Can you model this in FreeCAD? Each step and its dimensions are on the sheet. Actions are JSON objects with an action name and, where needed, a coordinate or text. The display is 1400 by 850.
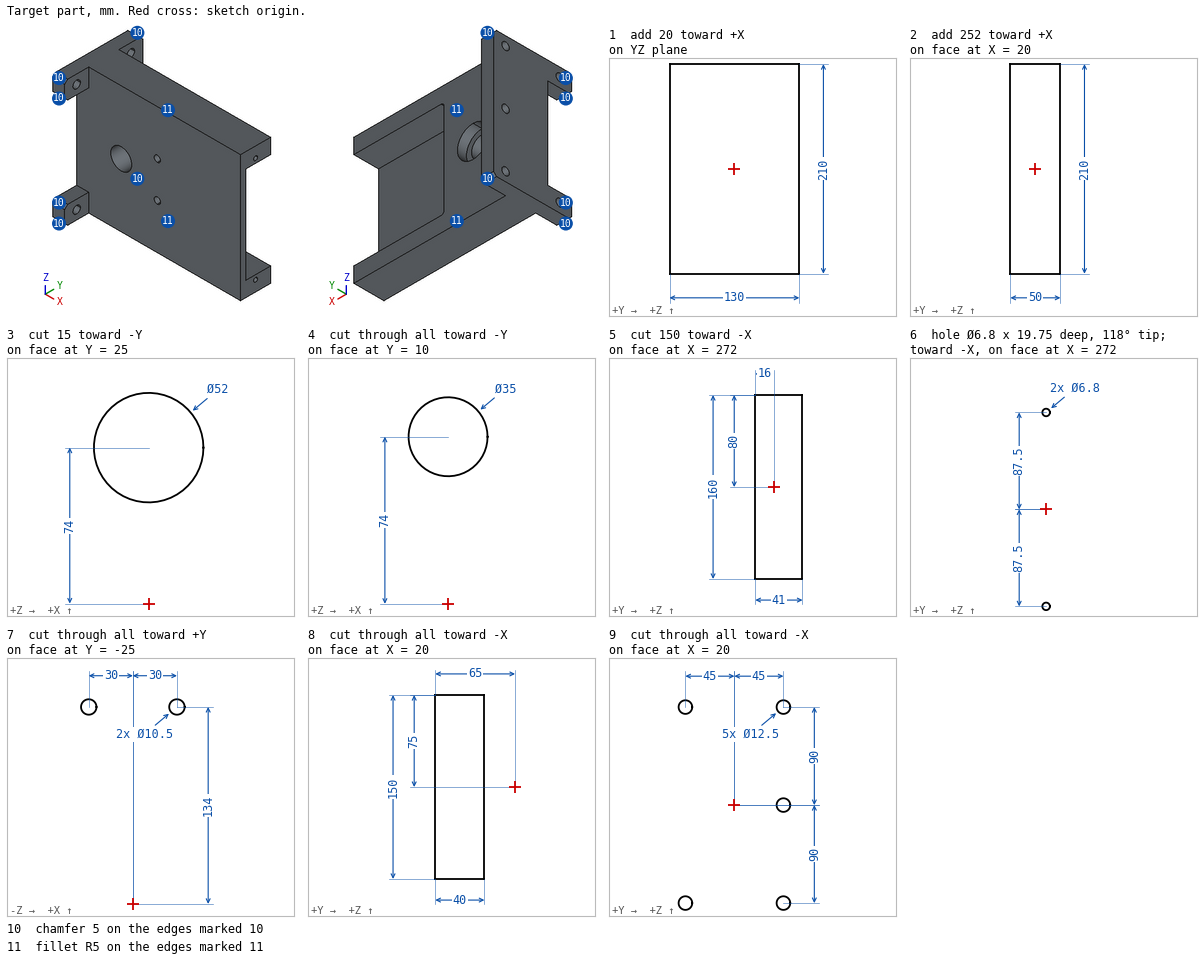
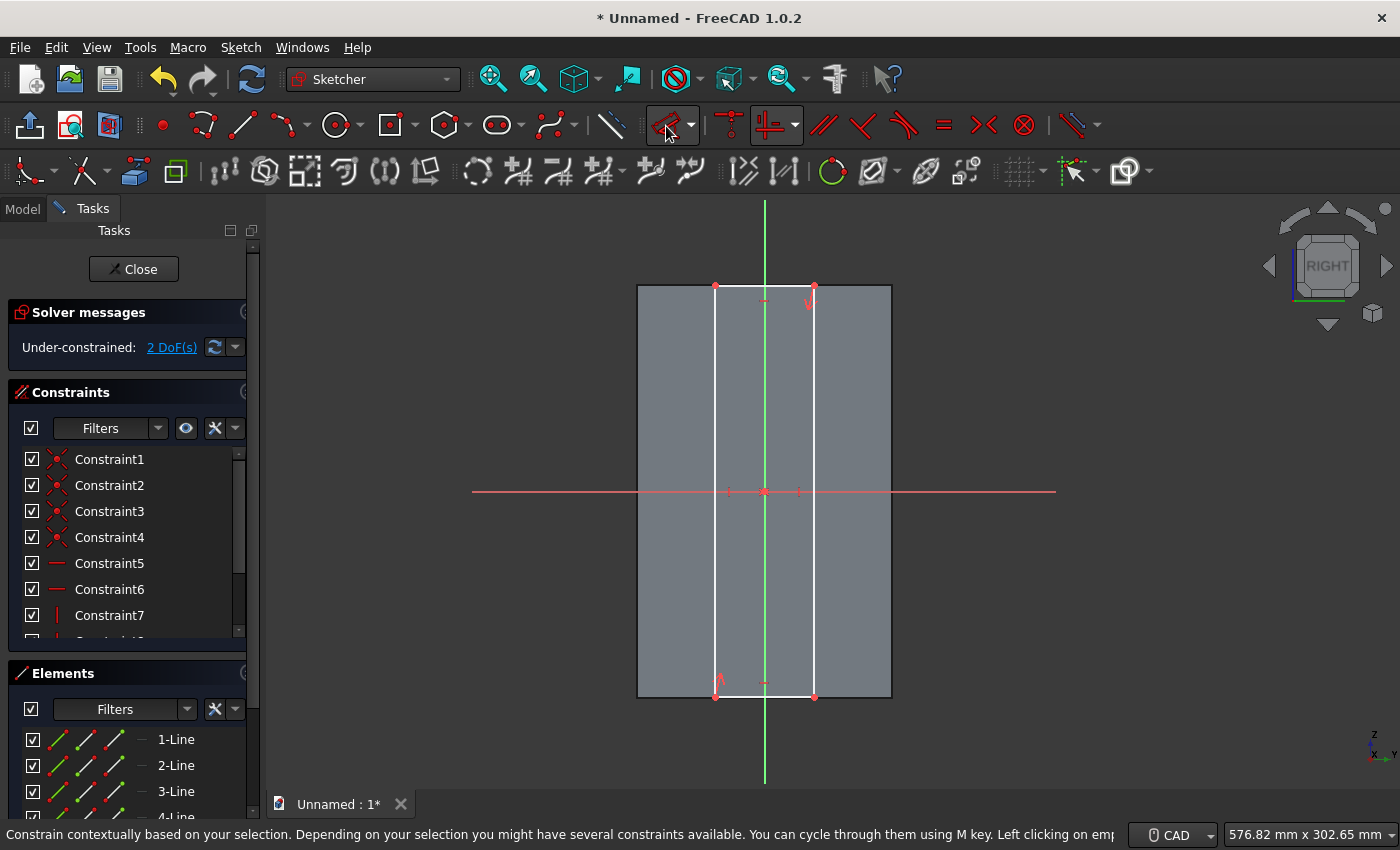
{"action": "left_click", "coordinate": [745, 697]}
{"action": "left_click", "coordinate": [742, 731]}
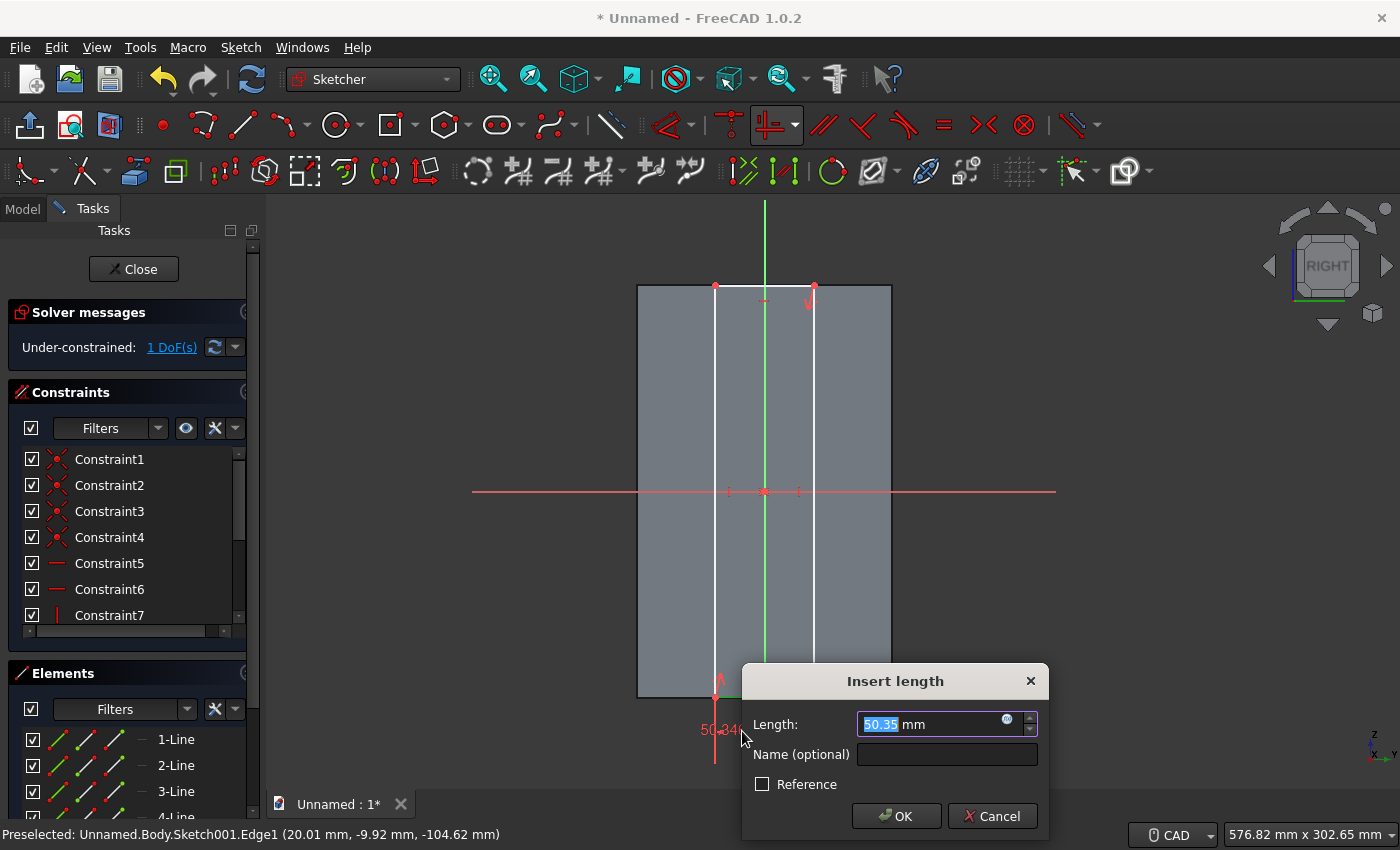
{"action": "type", "text": "50"}
{"action": "key", "text": "Return"}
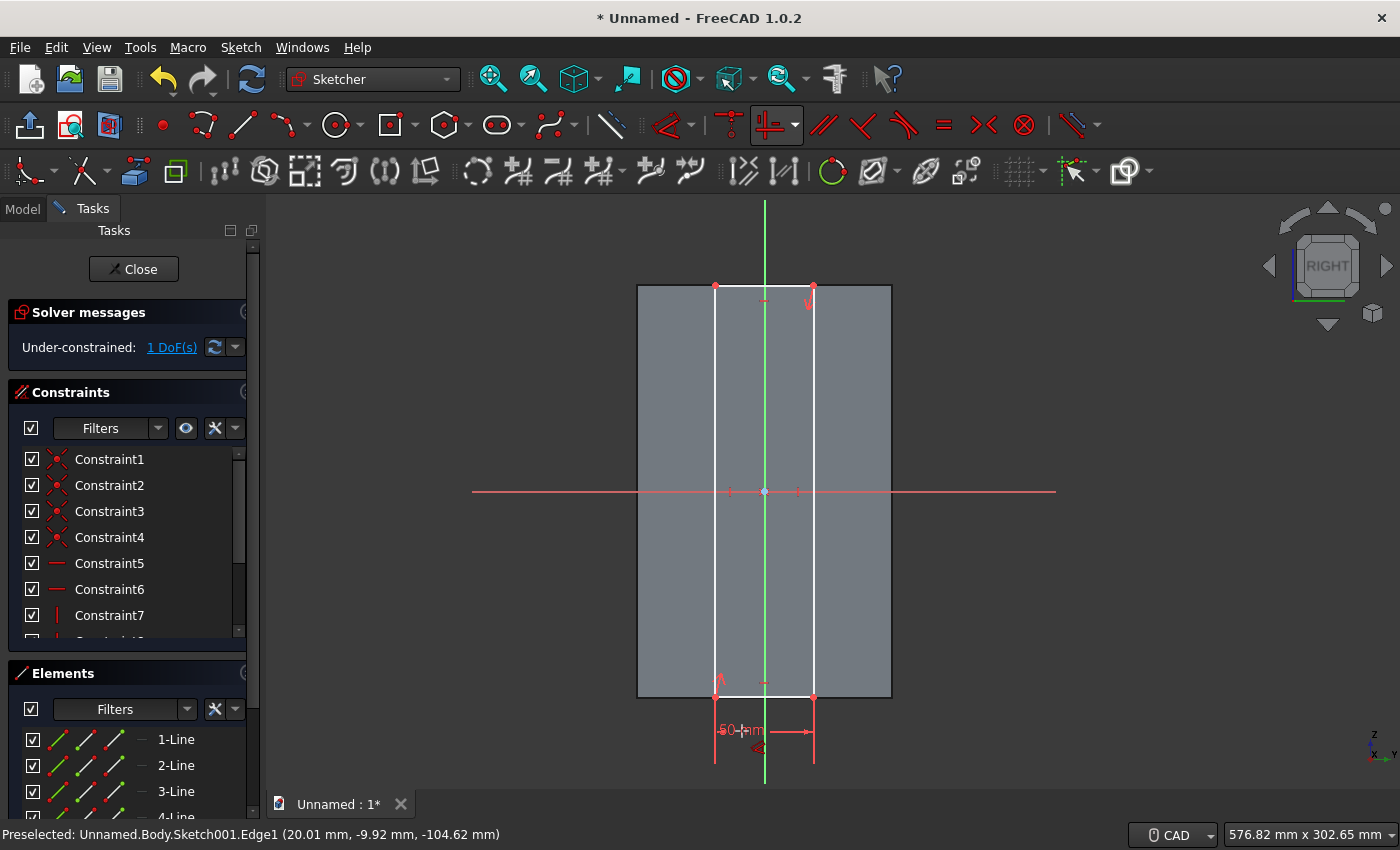
{"action": "left_click", "coordinate": [814, 574]}
{"action": "left_click", "coordinate": [848, 397]}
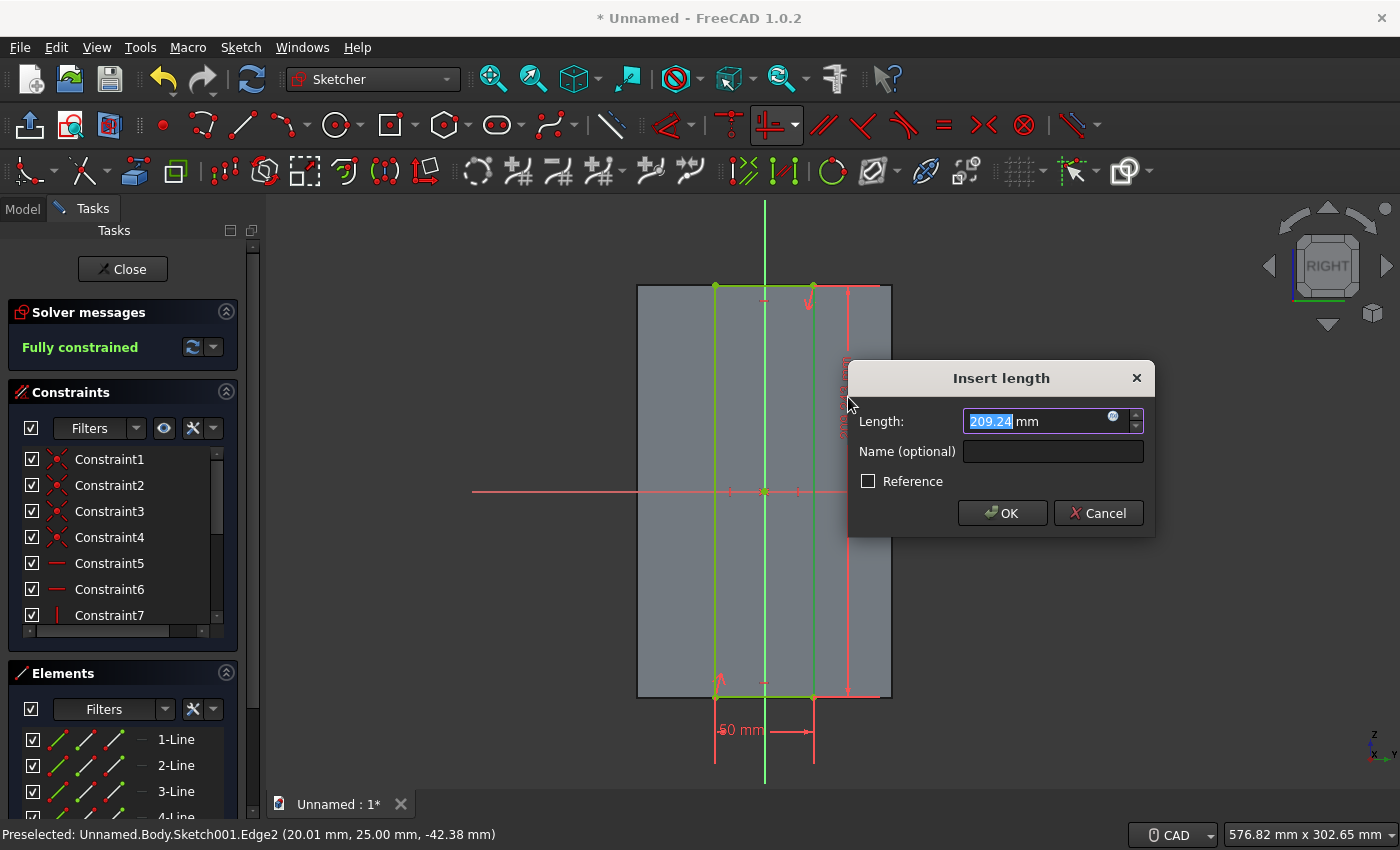
{"action": "type", "text": "210"}
{"action": "key", "text": "Return"}
{"action": "key", "text": "Escape"}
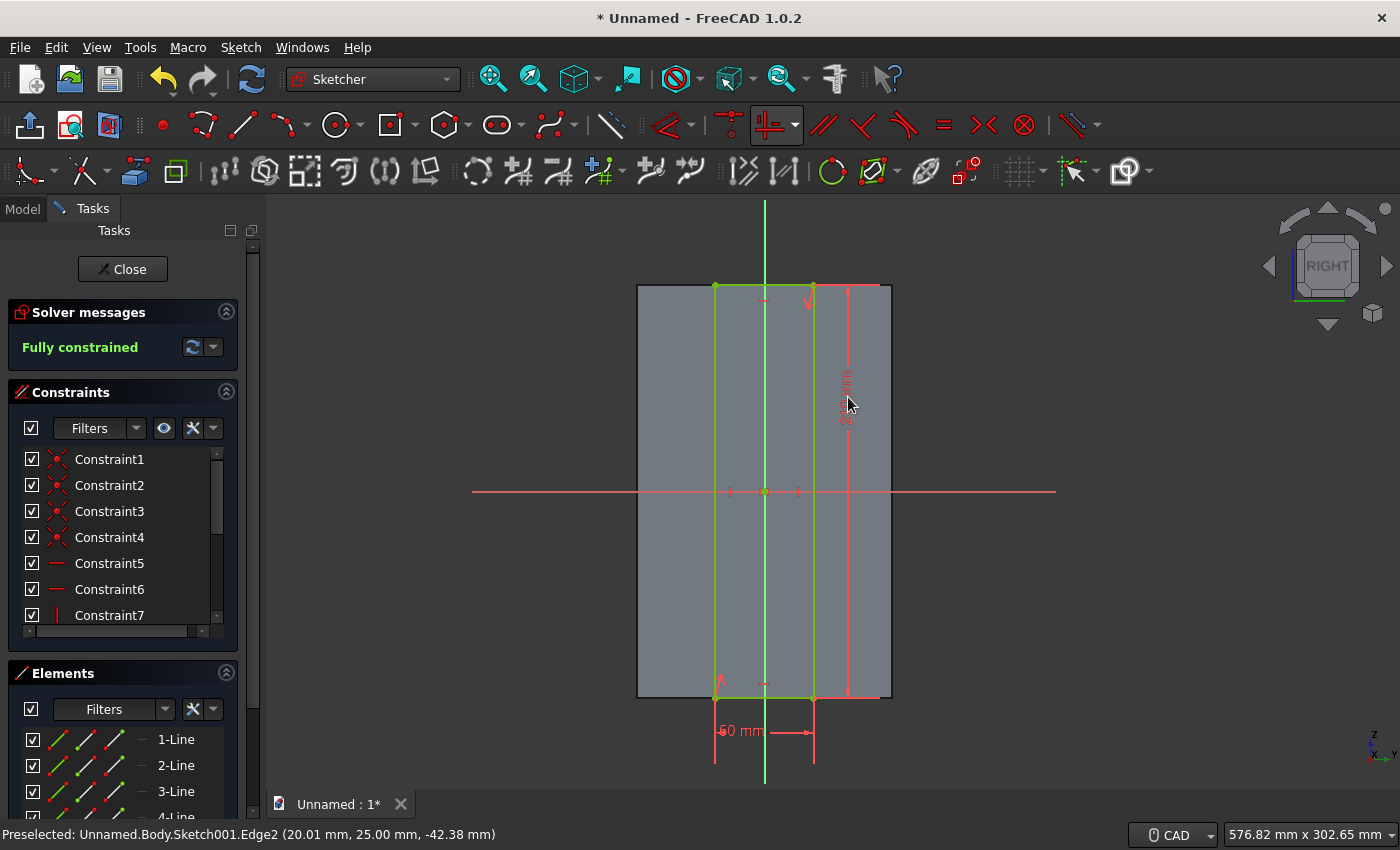
{"action": "left_click", "coordinate": [123, 269]}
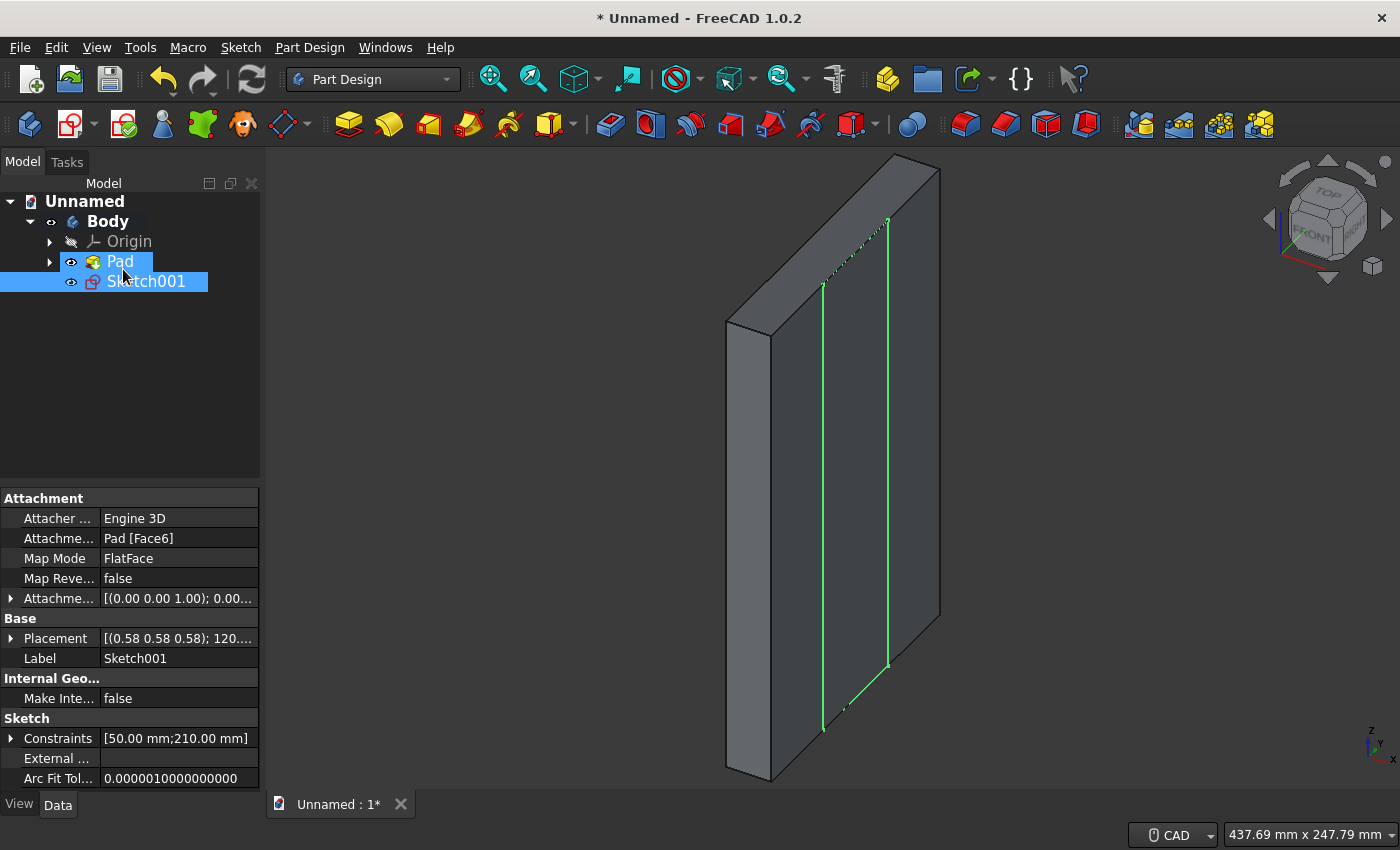
{"action": "left_click", "coordinate": [350, 124]}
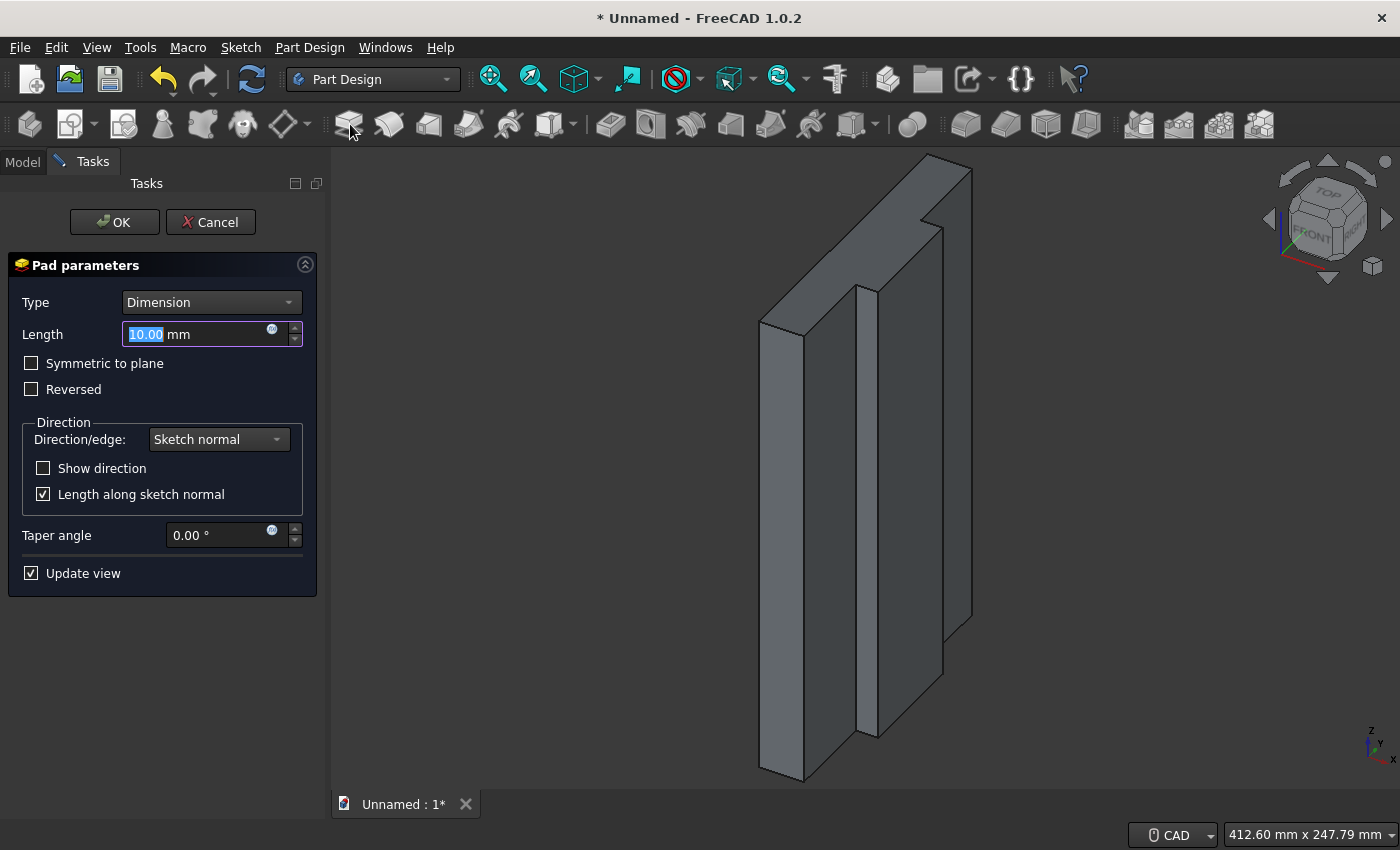
{"action": "type", "text": "252"}
{"action": "key", "text": "Tab"}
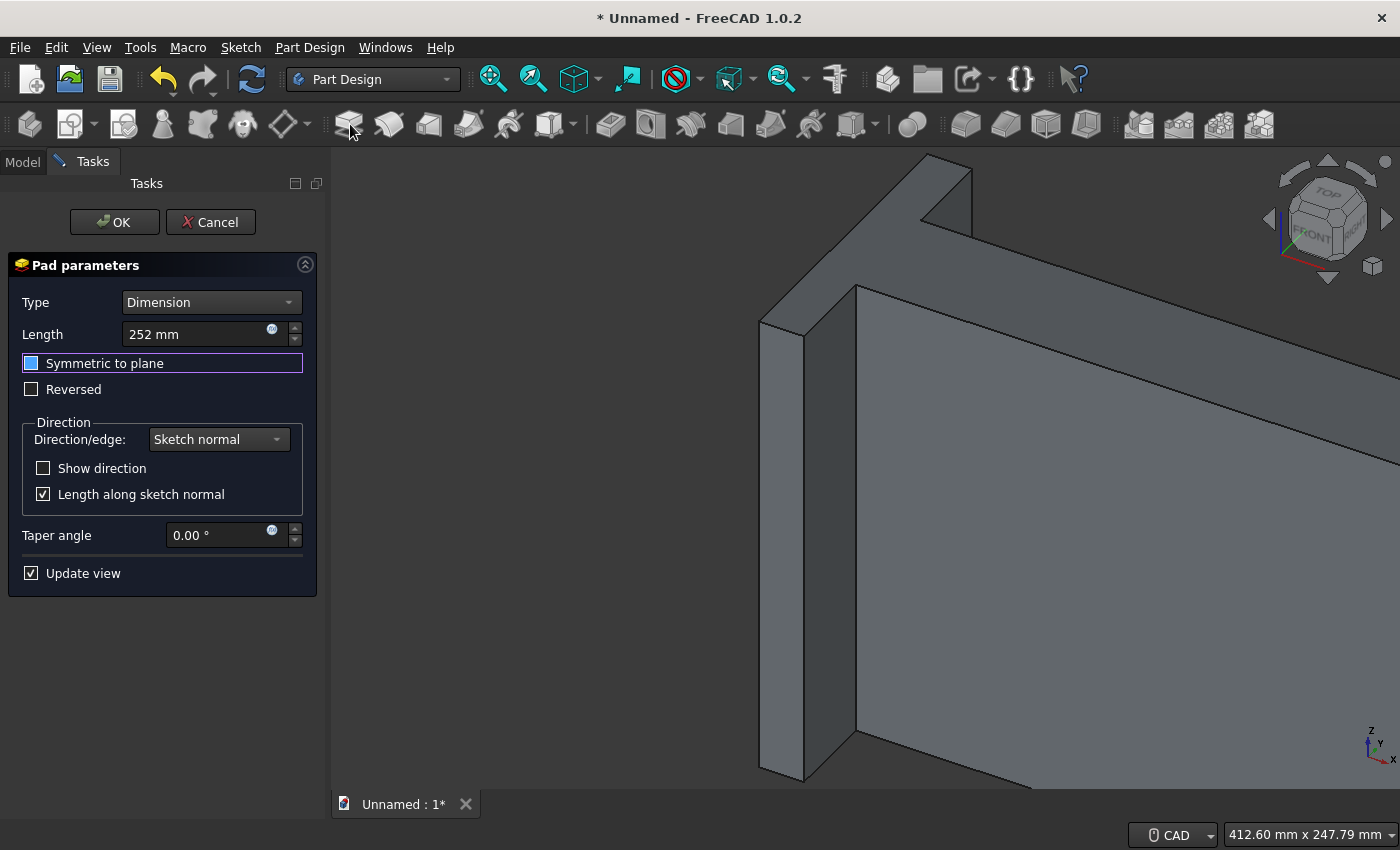
{"action": "left_click", "coordinate": [115, 222]}